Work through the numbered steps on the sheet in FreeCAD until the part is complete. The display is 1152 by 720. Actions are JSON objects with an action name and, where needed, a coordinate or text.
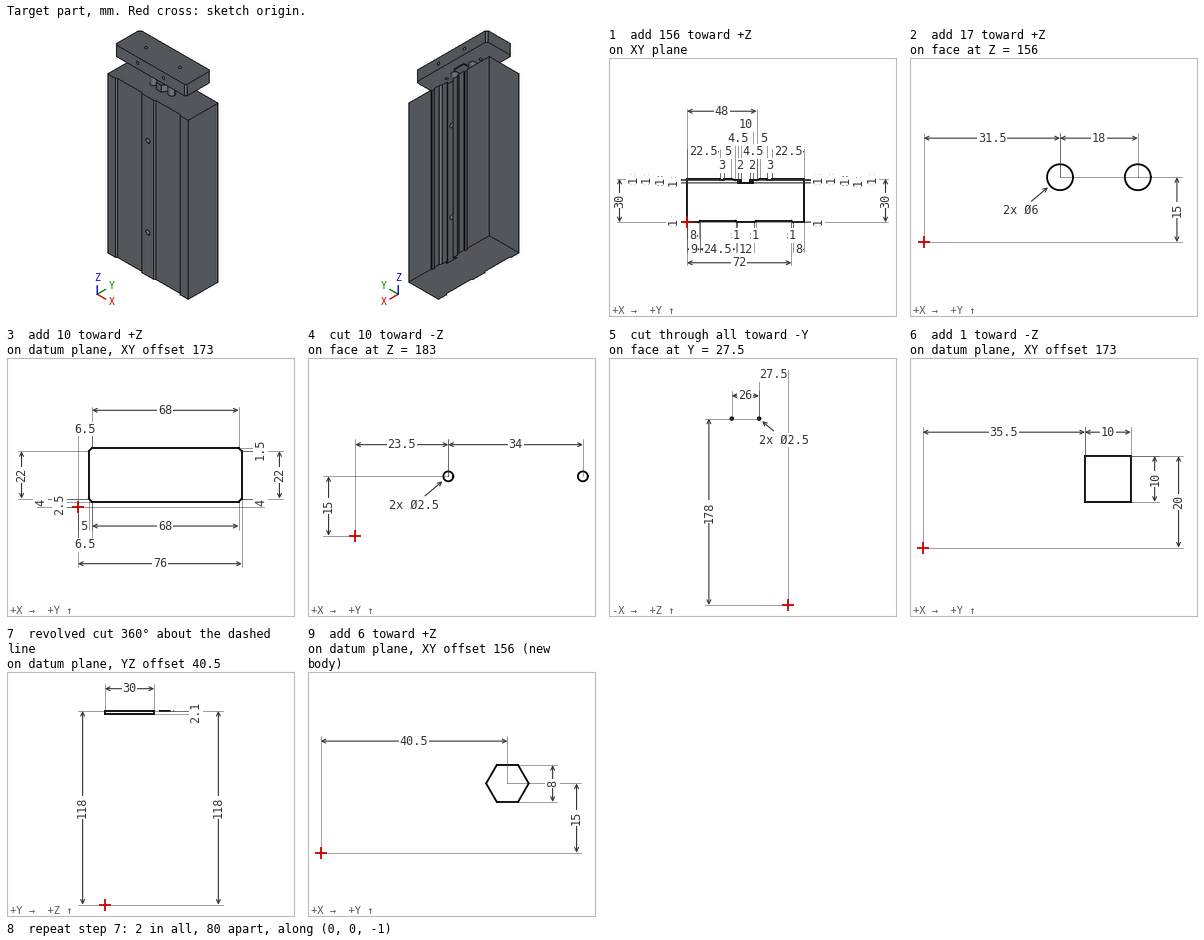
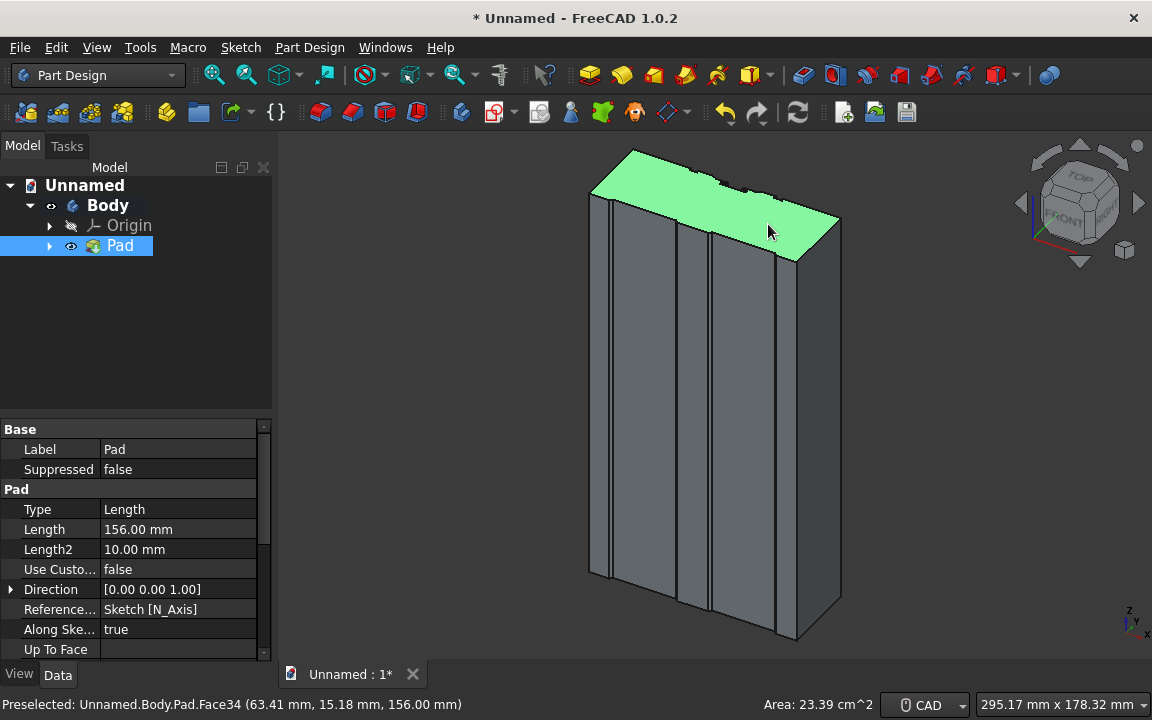
{"action": "left_click", "coordinate": [494, 112]}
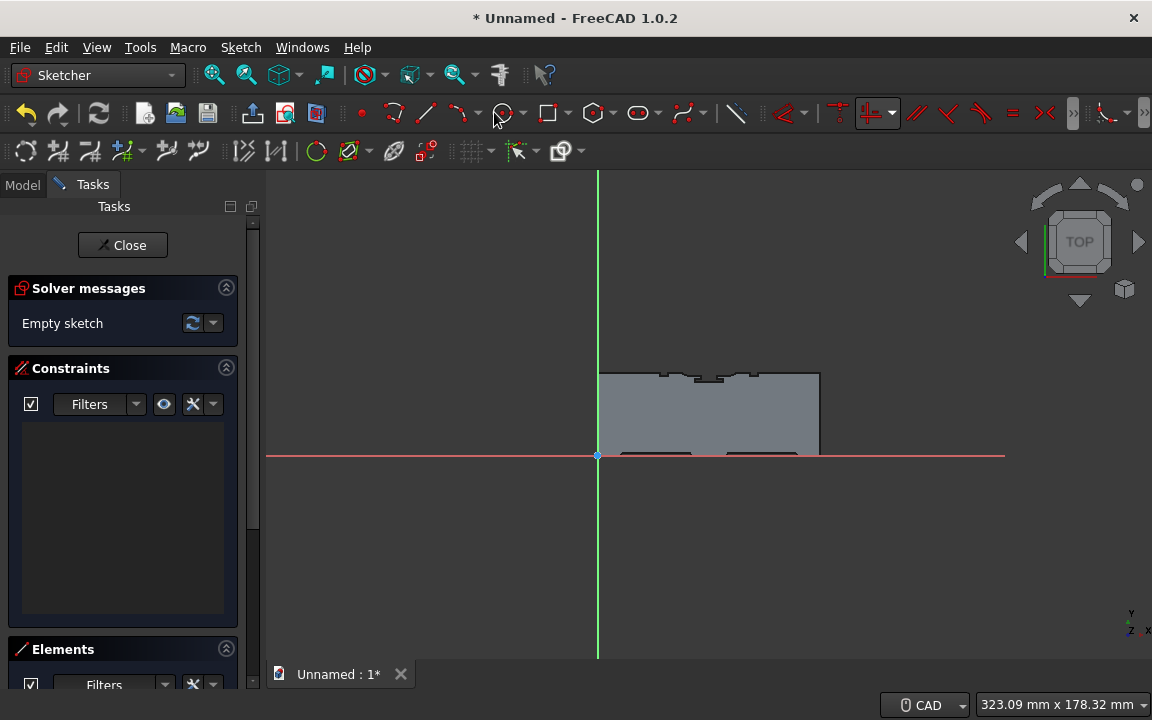
{"action": "scroll", "coordinate": [683, 438], "scroll_direction": "up", "scroll_amount": 6}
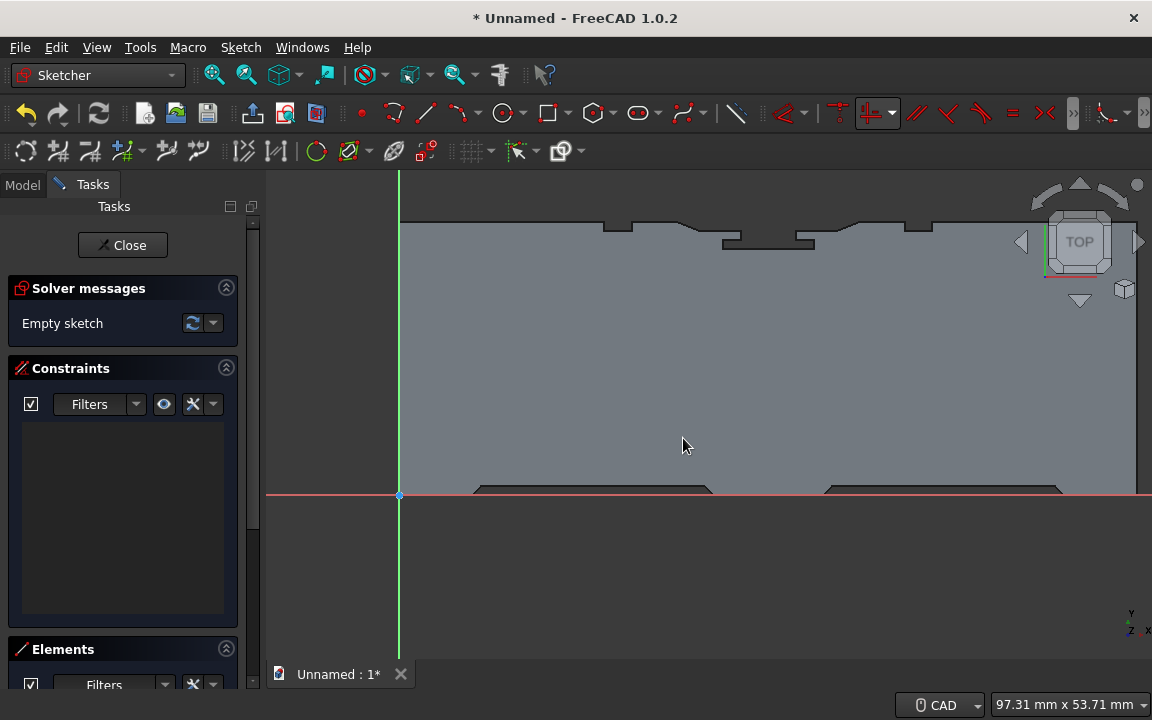
{"action": "key", "text": "g c"}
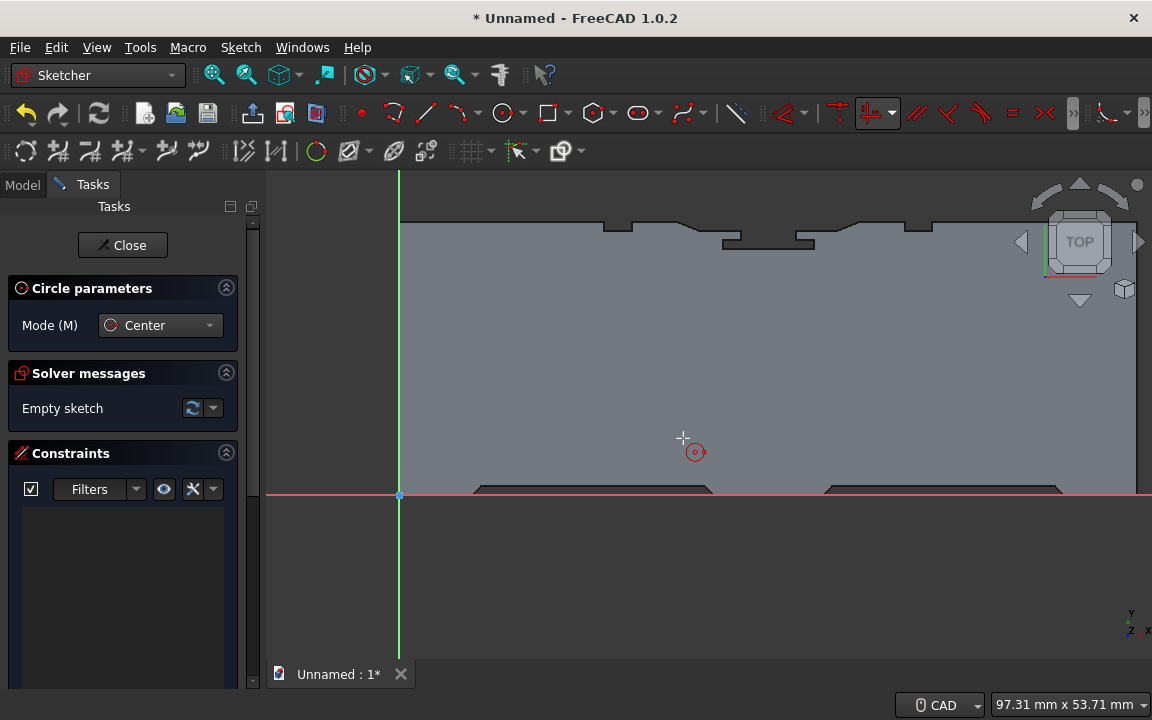
{"action": "left_click", "coordinate": [686, 359]}
{"action": "mouse_move", "coordinate": [706, 339]}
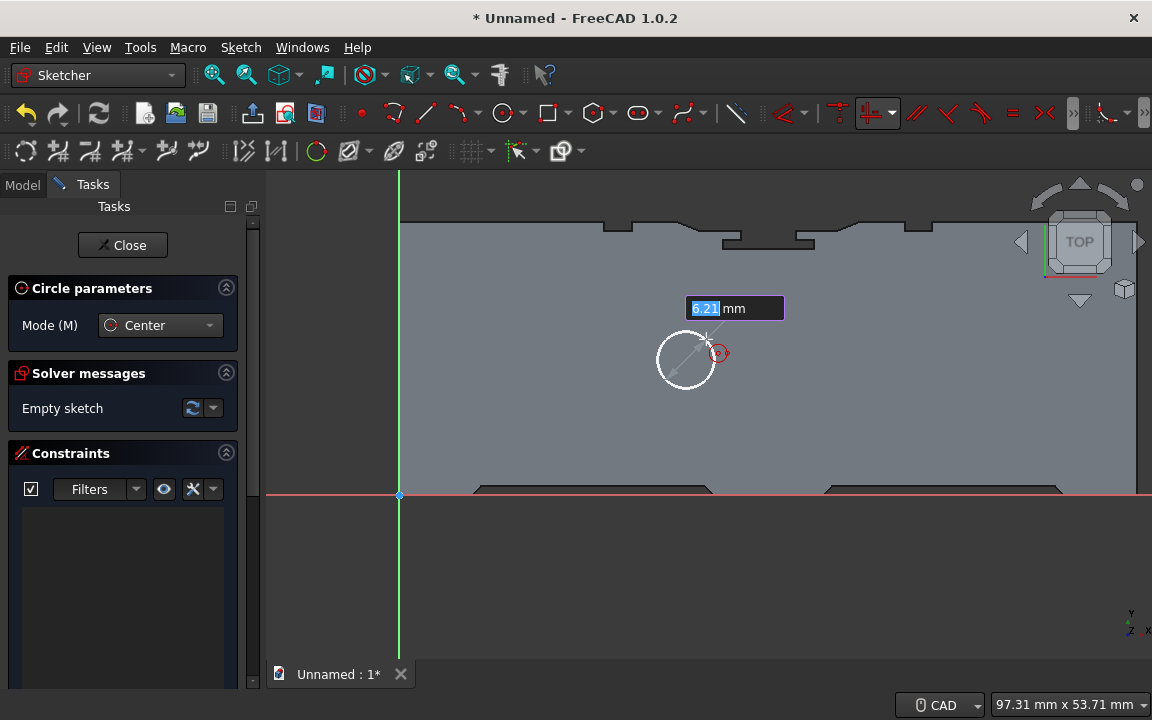
{"action": "type", "text": "6"}
{"action": "key", "text": "Return"}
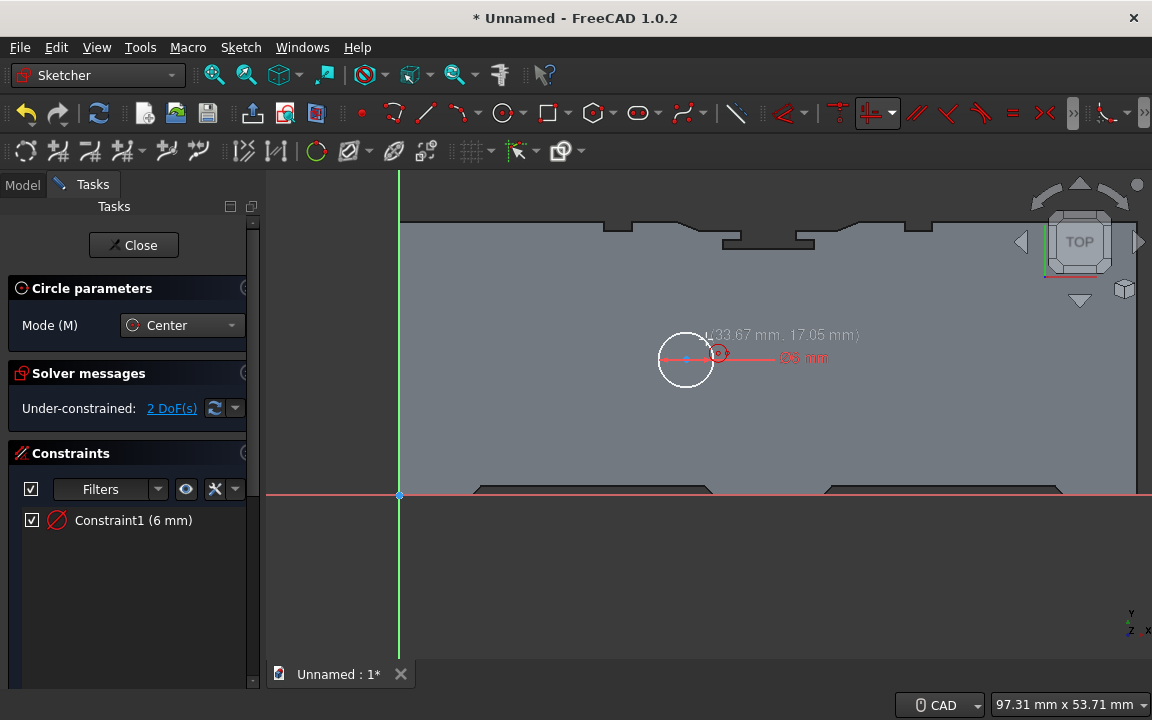
{"action": "left_click", "coordinate": [850, 359]}
{"action": "mouse_move", "coordinate": [869, 339]}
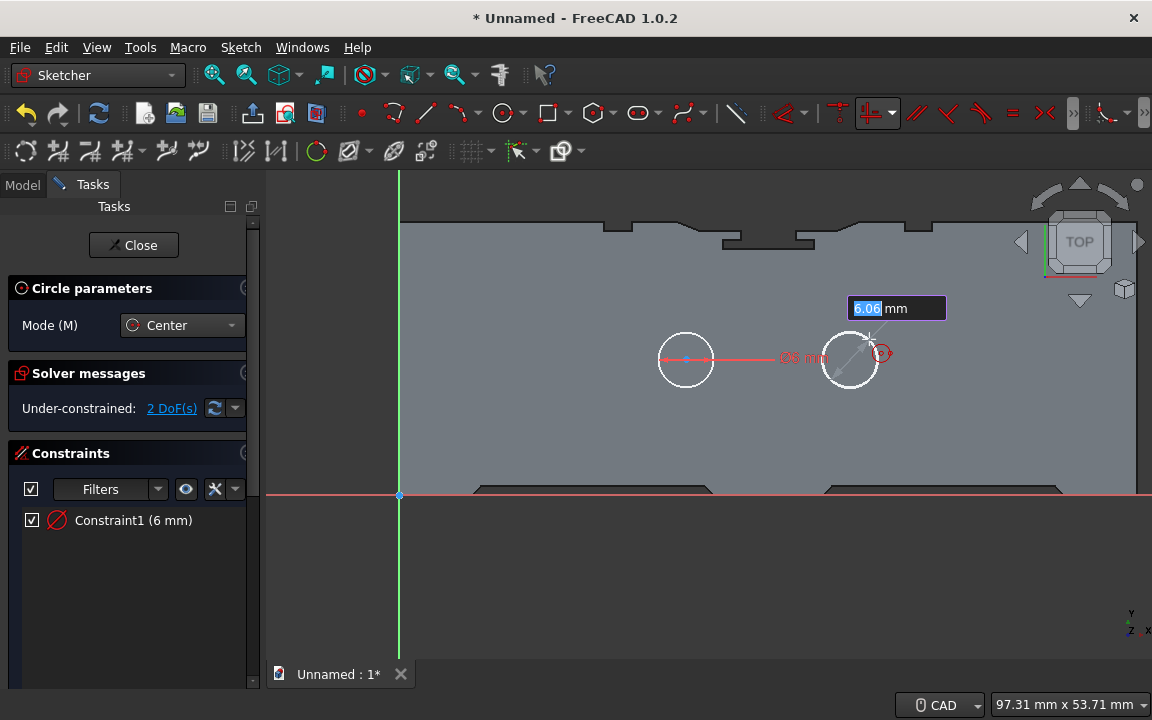
{"action": "type", "text": "6"}
{"action": "key", "text": "Return"}
{"action": "key", "text": "Escape"}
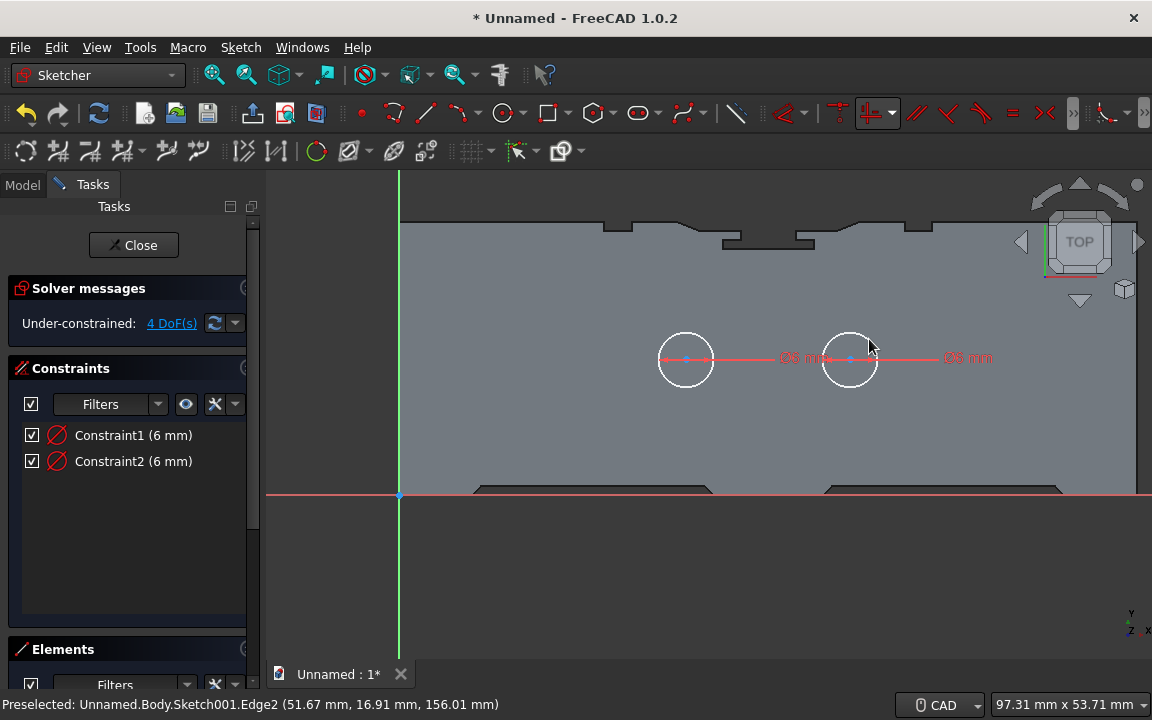
{"action": "left_click", "coordinate": [686, 360]}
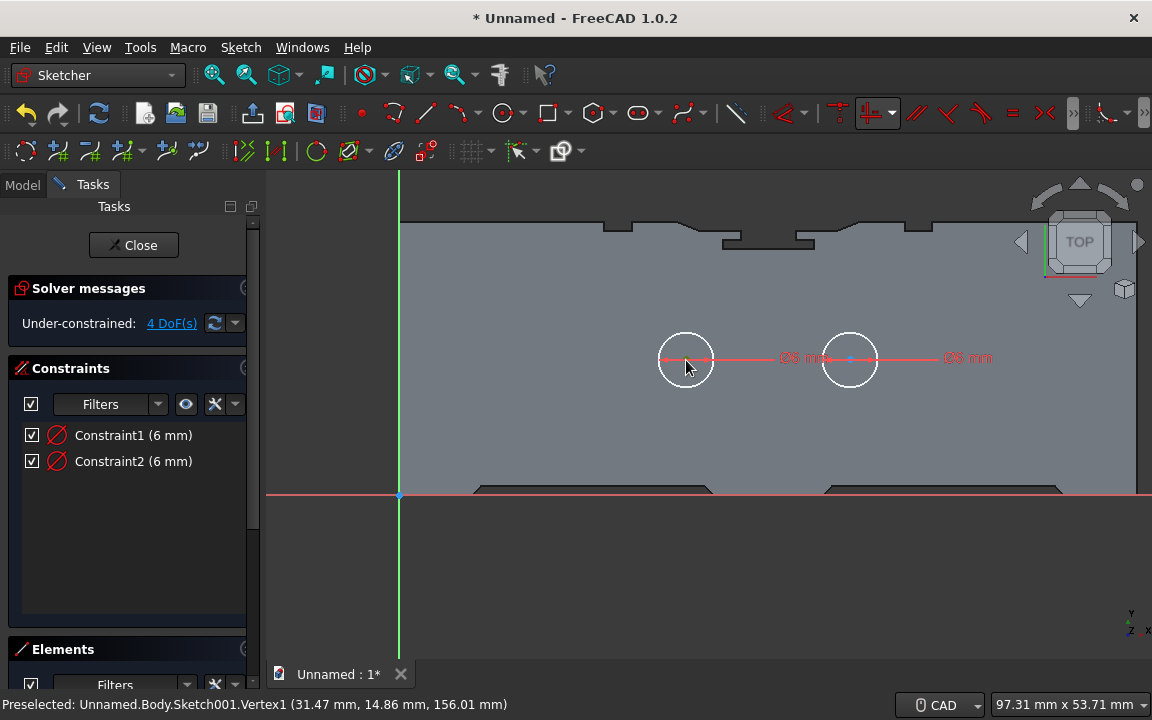
{"action": "left_click", "coordinate": [850, 360]}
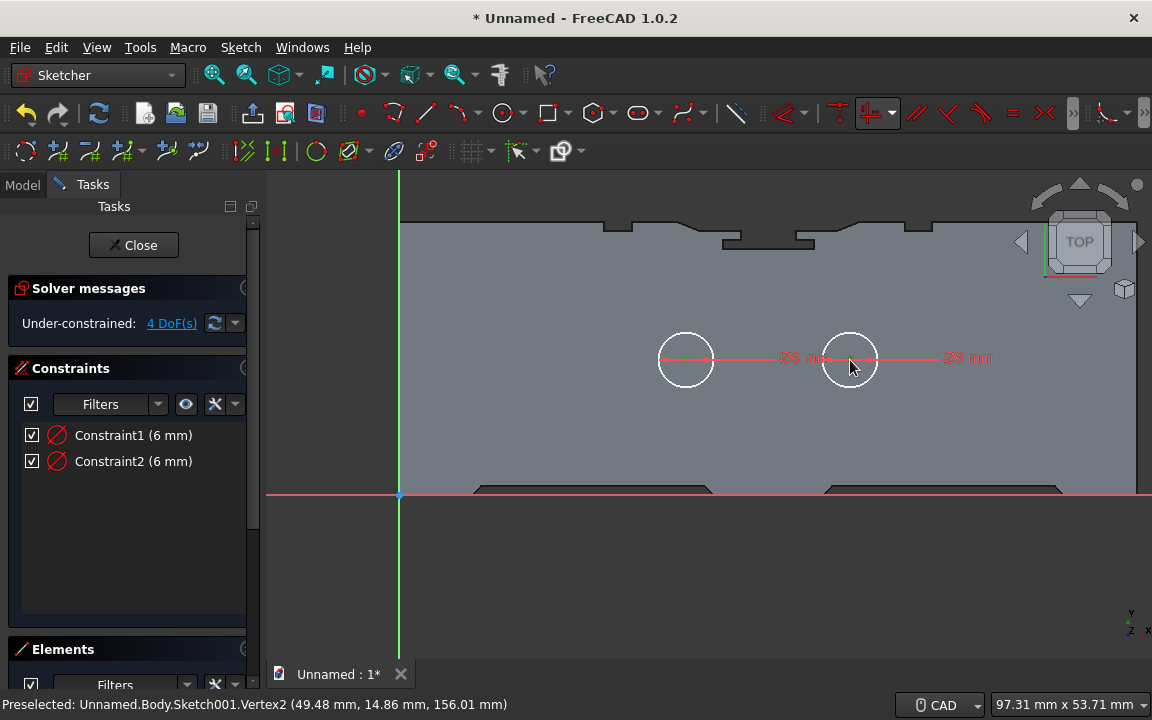
{"action": "key", "text": "h"}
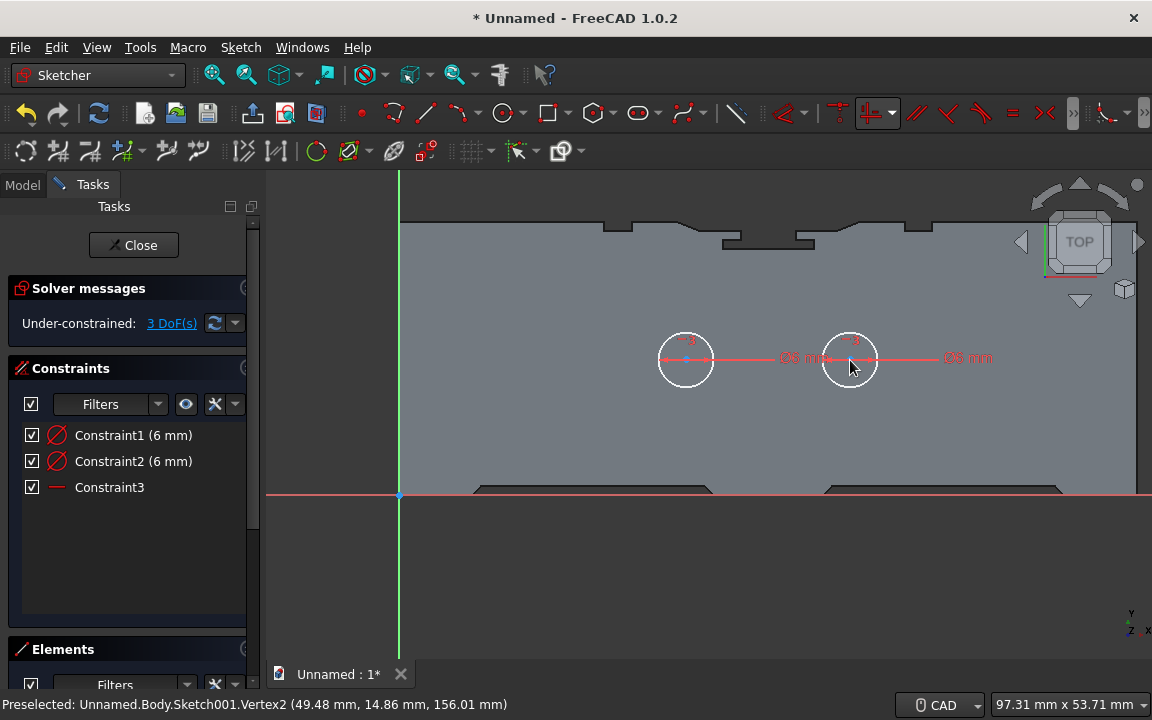
{"action": "key", "text": "d"}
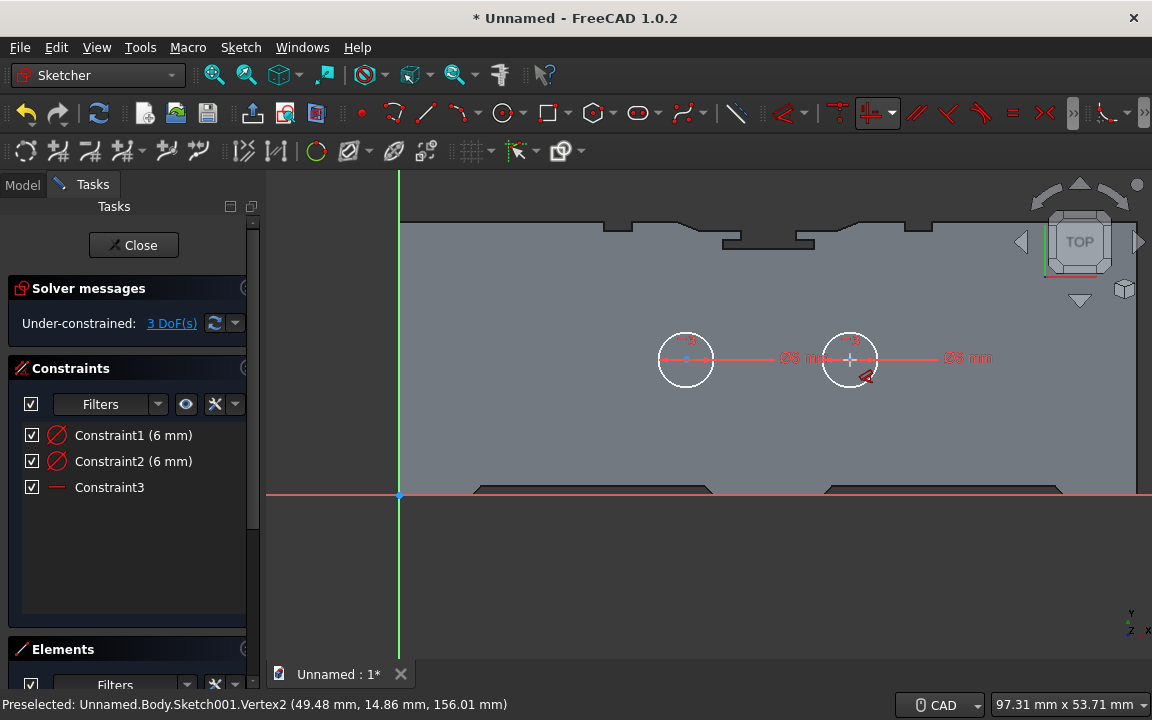
{"action": "left_click", "coordinate": [686, 360]}
{"action": "left_click", "coordinate": [365, 428]}